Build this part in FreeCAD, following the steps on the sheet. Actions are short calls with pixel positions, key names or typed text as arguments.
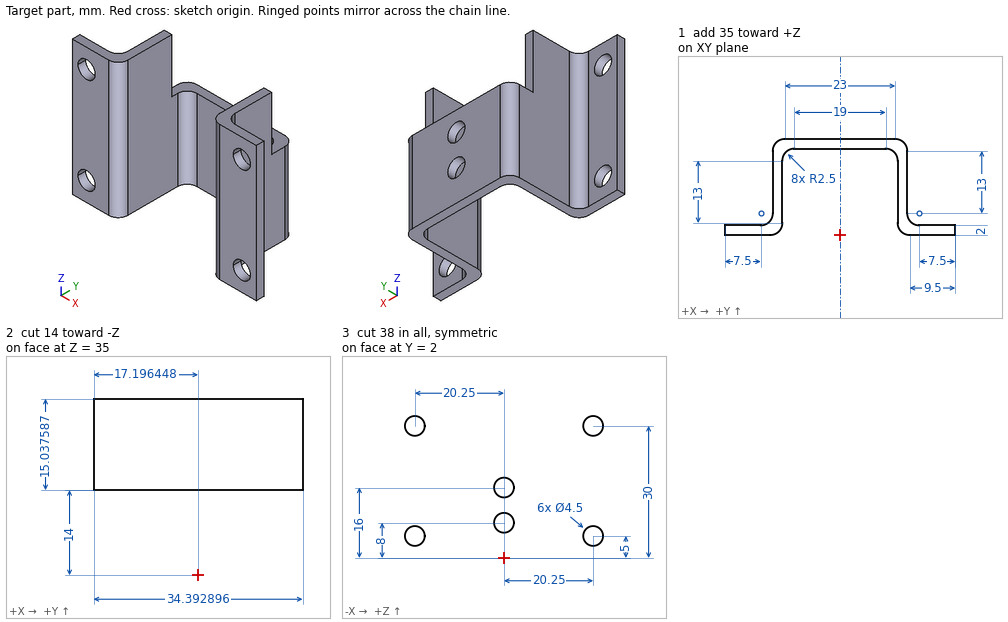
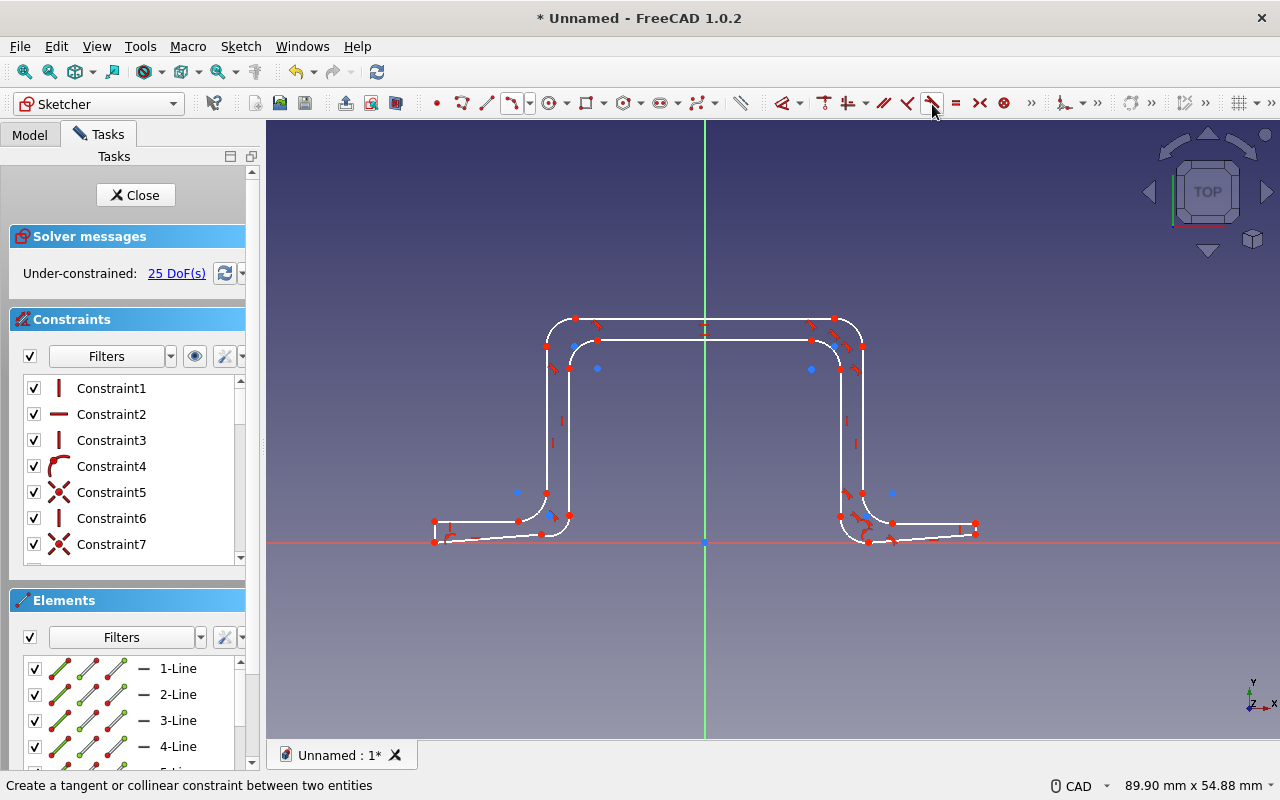
click(757, 319)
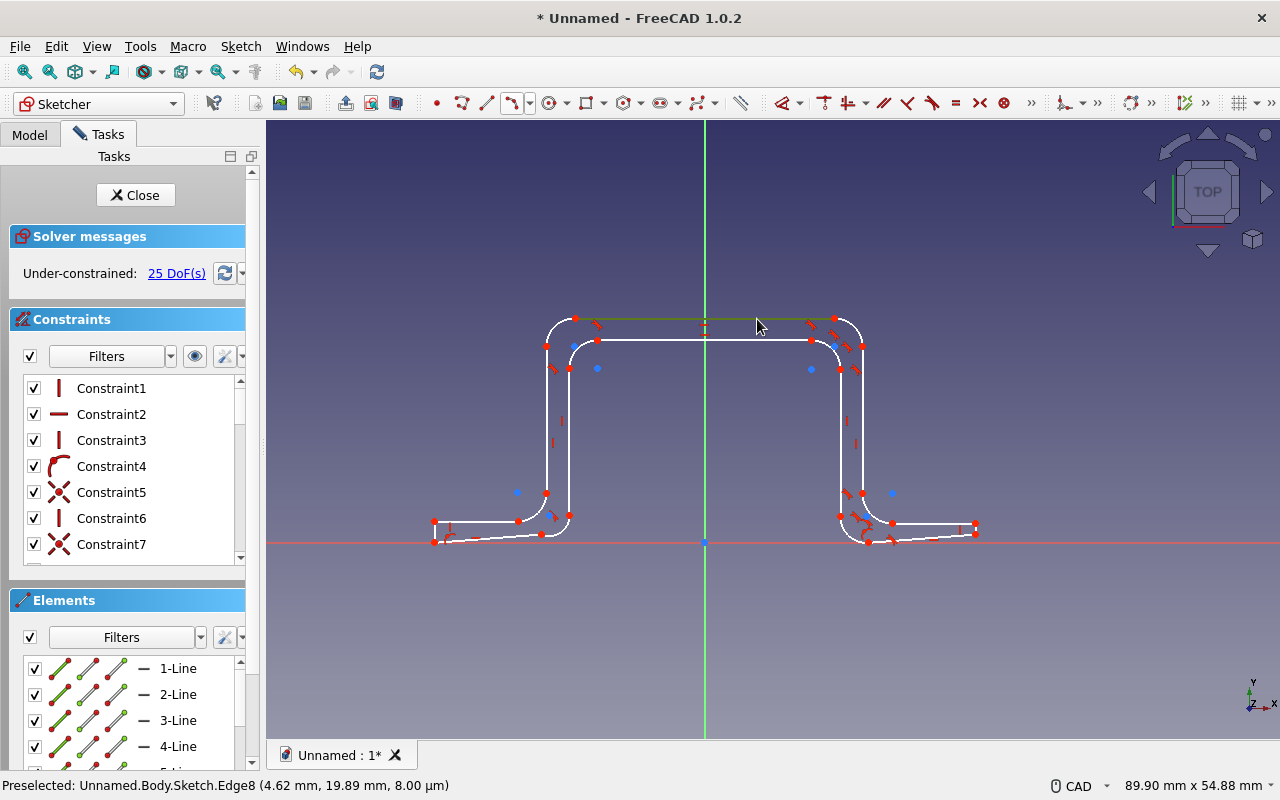
click(562, 321)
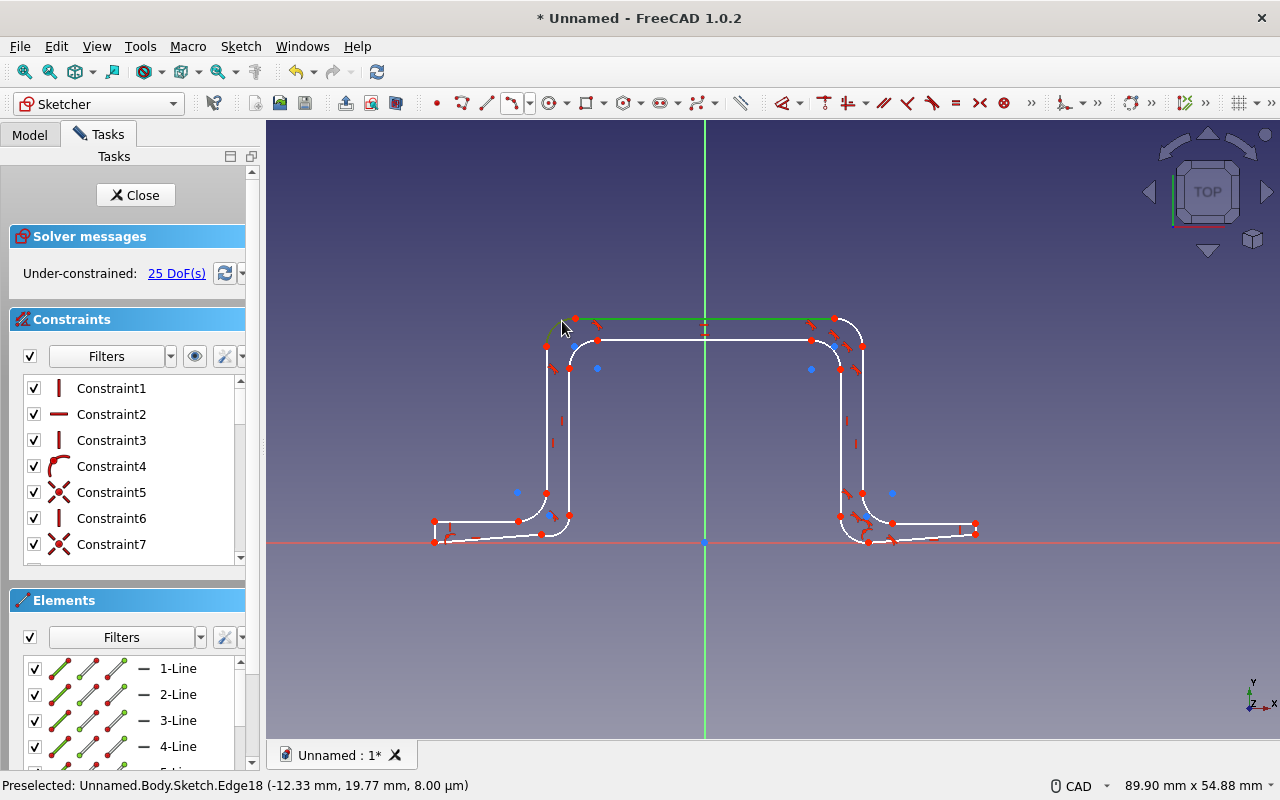
click(932, 104)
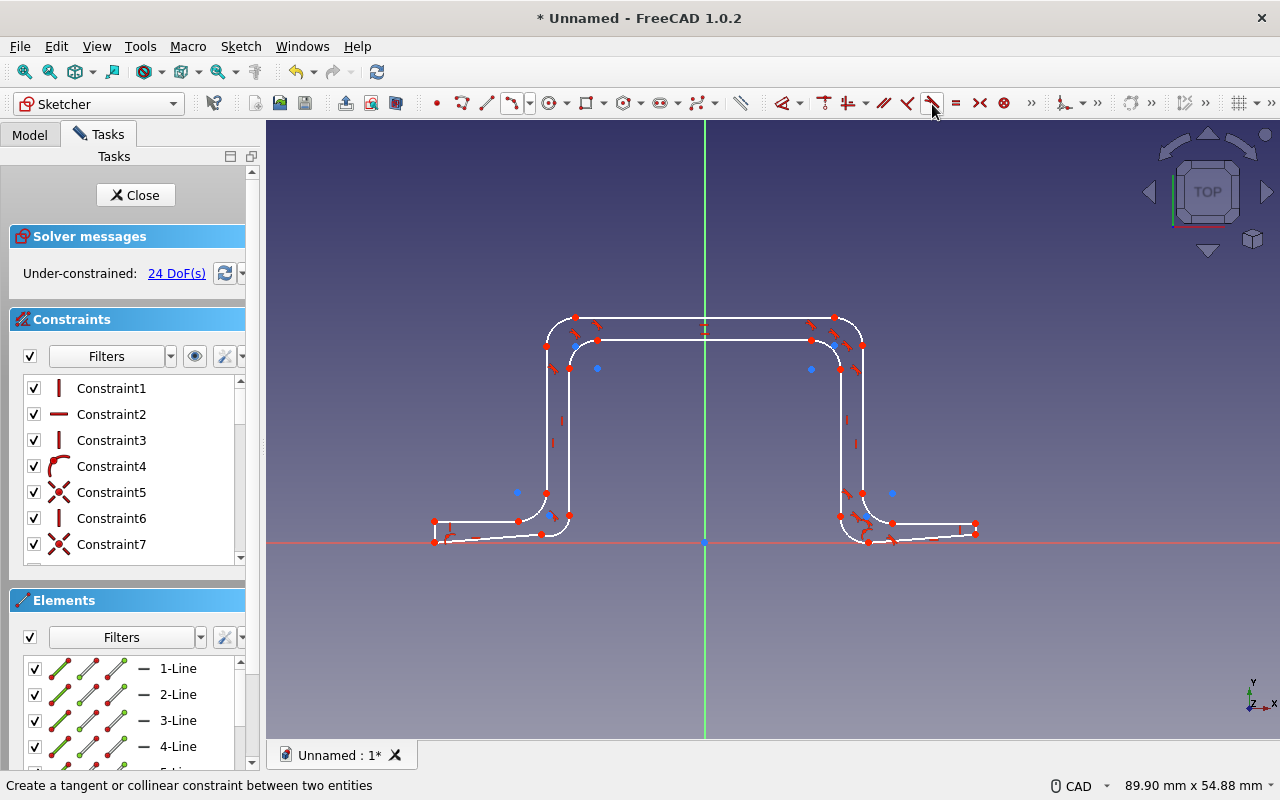
click(547, 391)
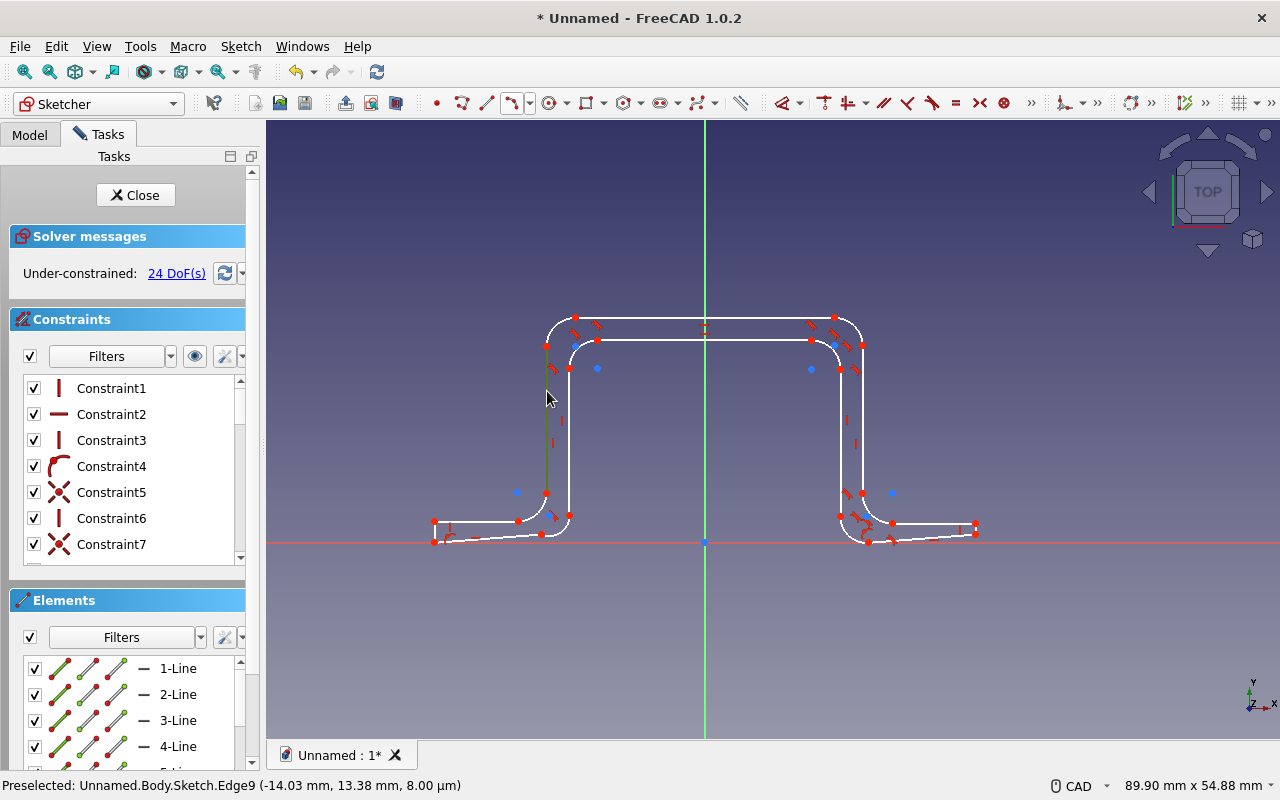
click(562, 321)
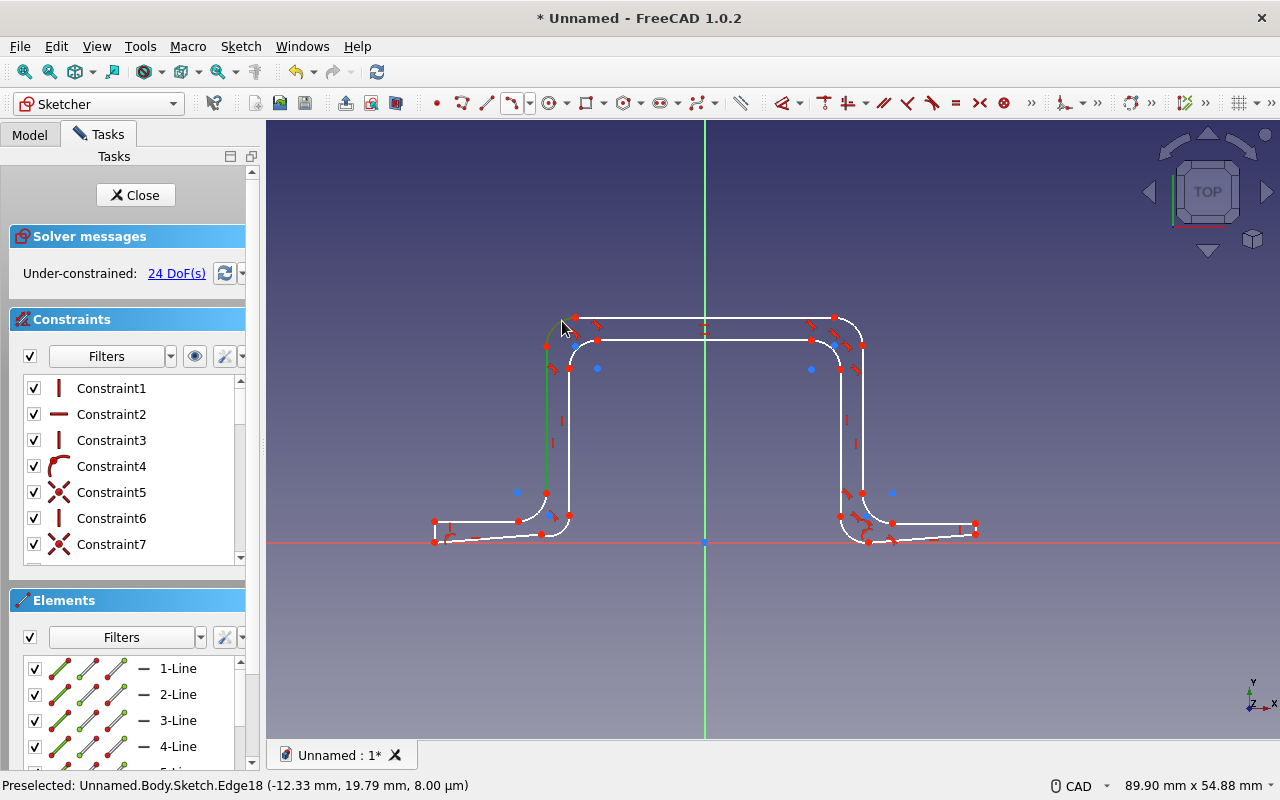
click(932, 104)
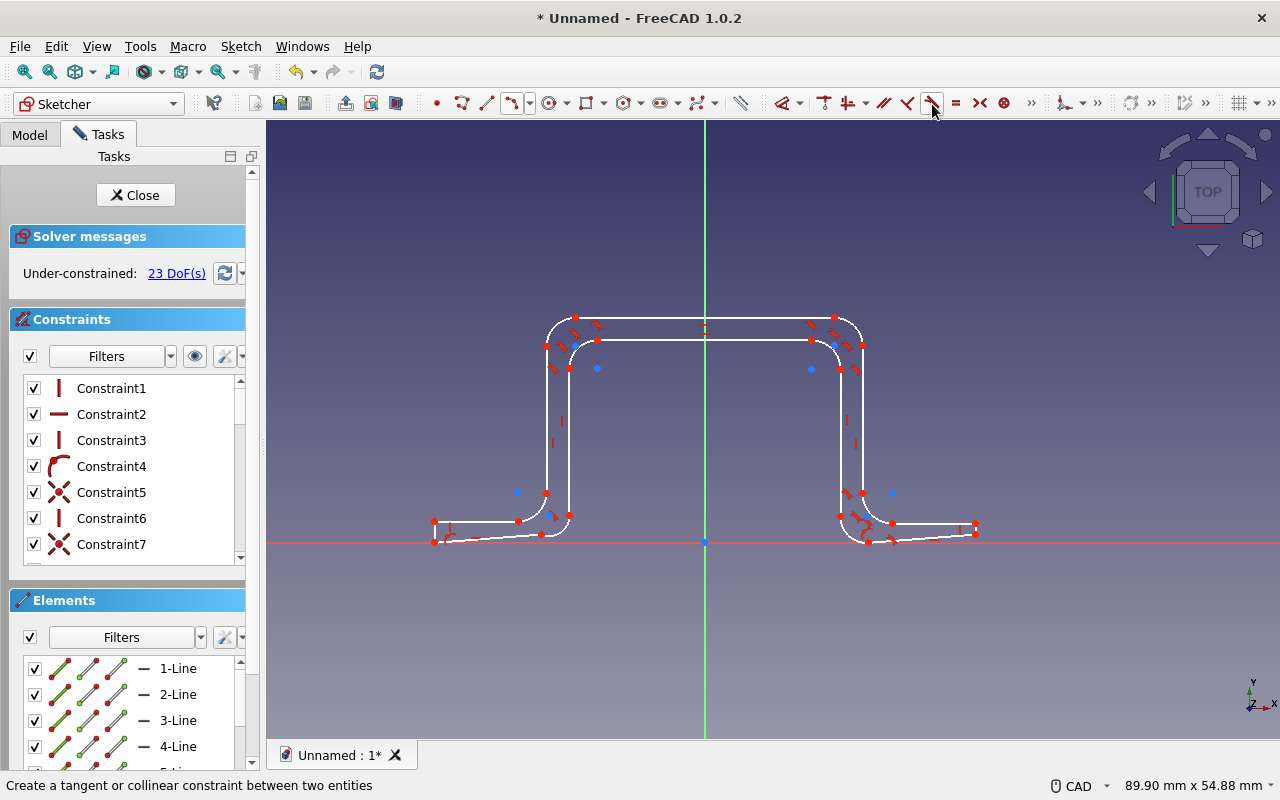
click(547, 391)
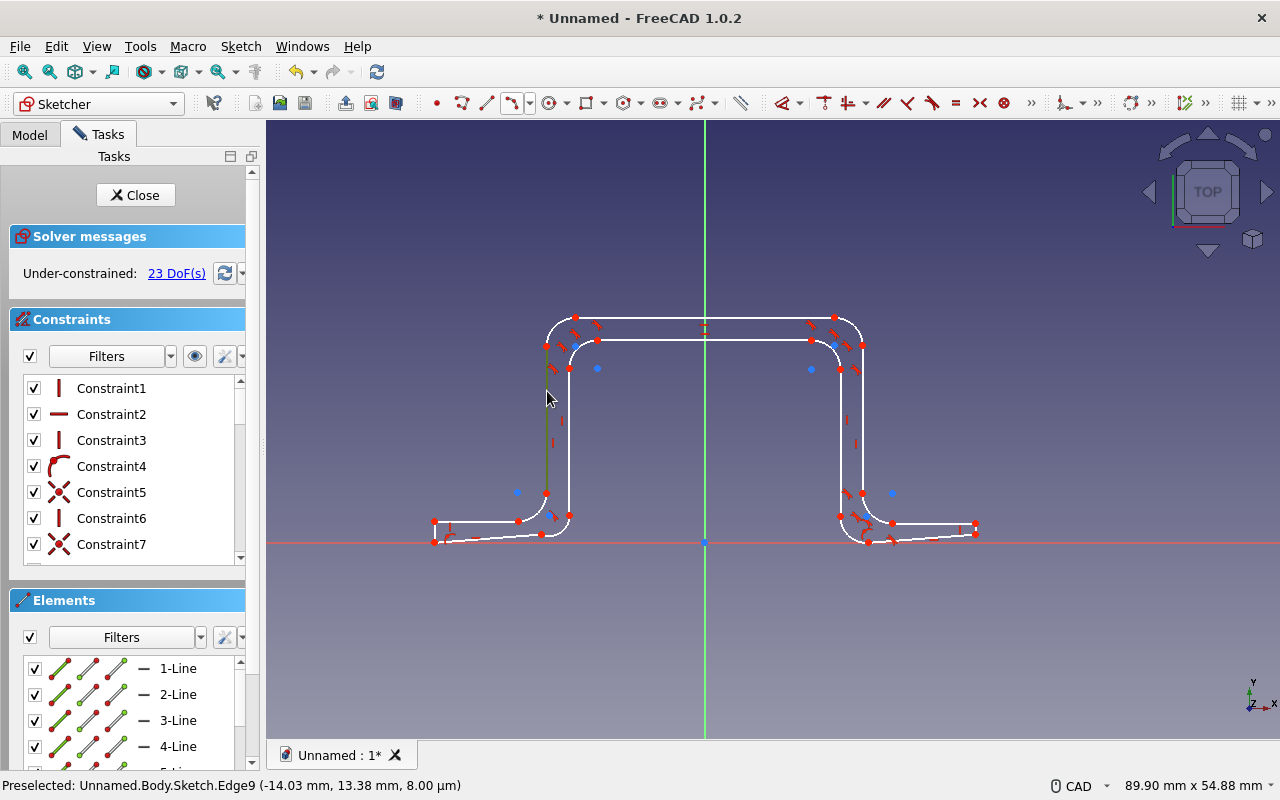
click(531, 518)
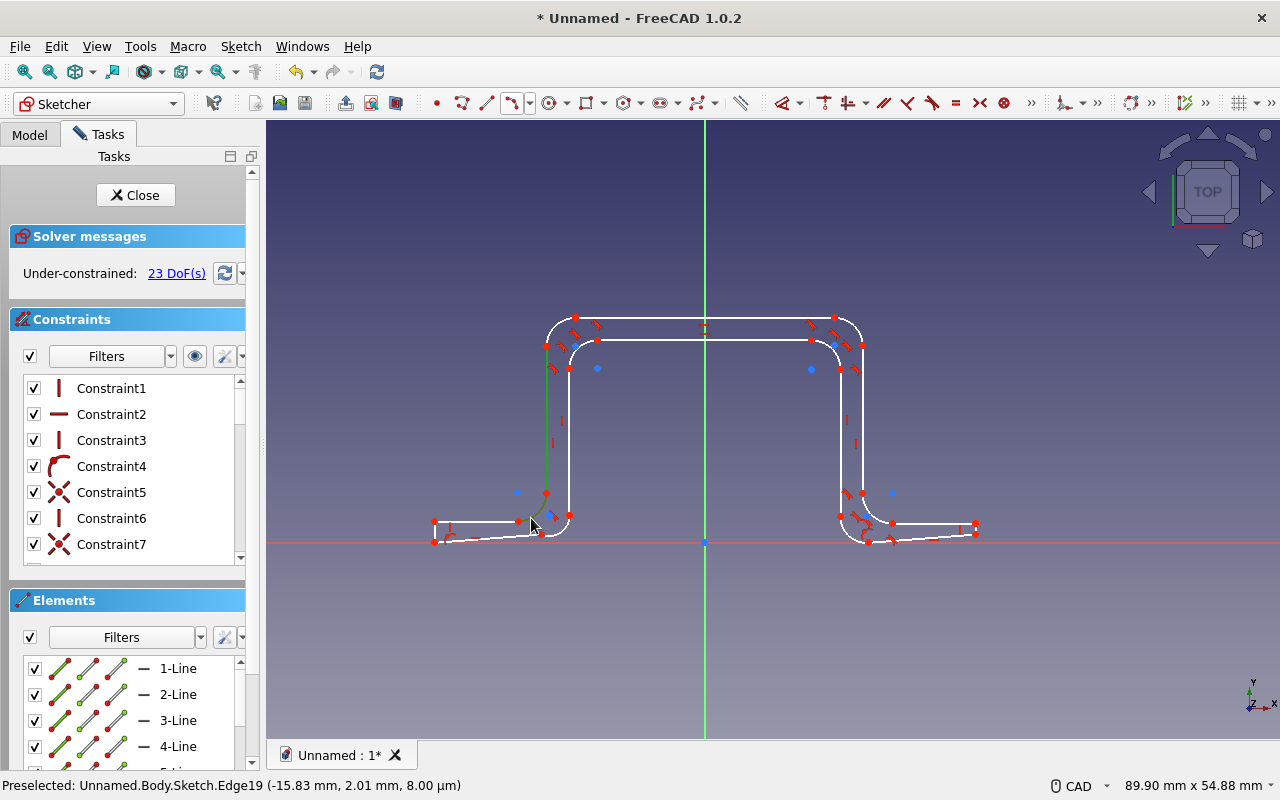
key(t)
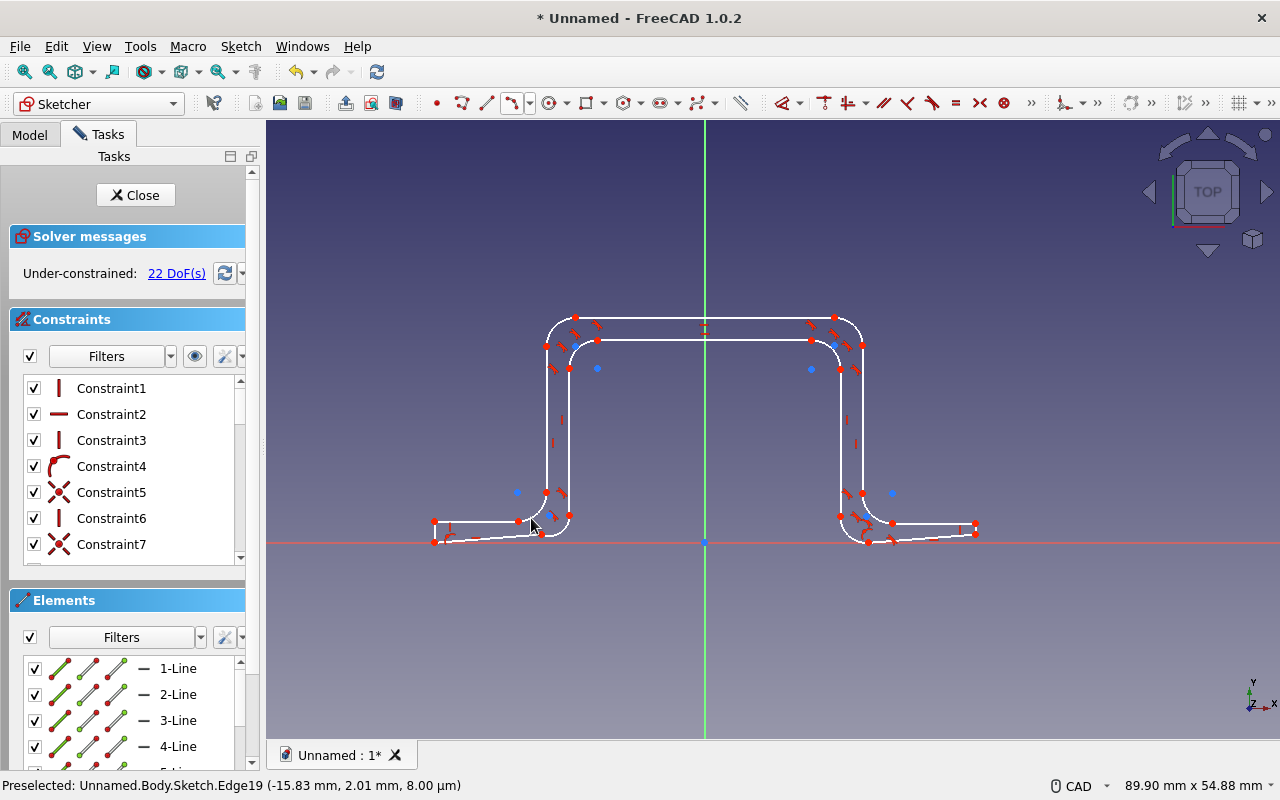
click(493, 522)